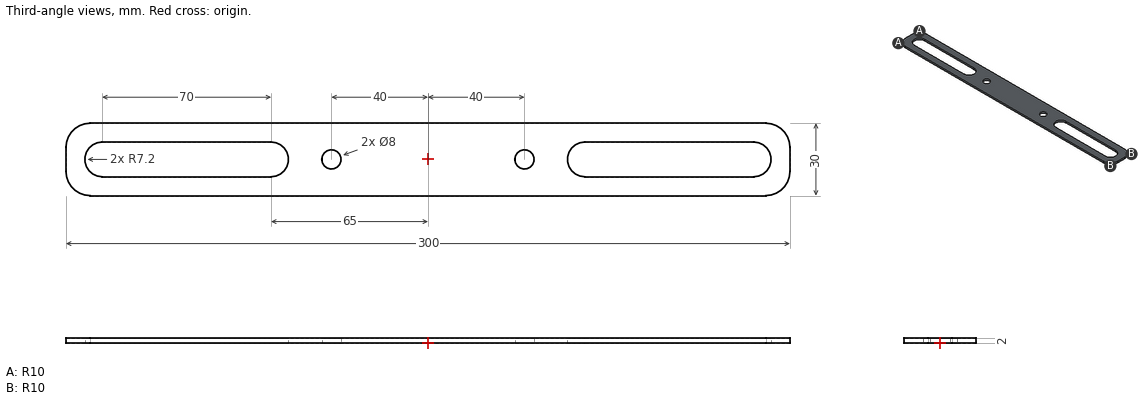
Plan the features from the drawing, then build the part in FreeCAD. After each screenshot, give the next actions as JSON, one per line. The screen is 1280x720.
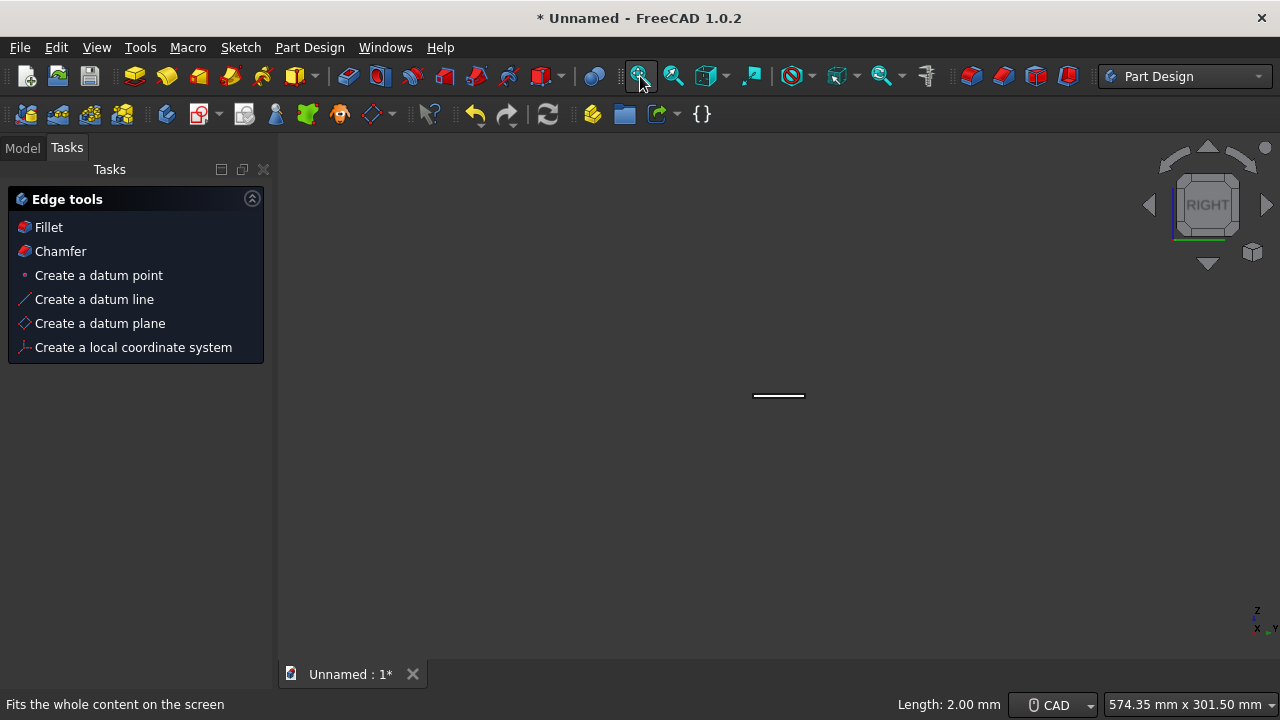
{"action": "scroll", "coordinate": [805, 395], "scroll_direction": "up", "scroll_amount": 13}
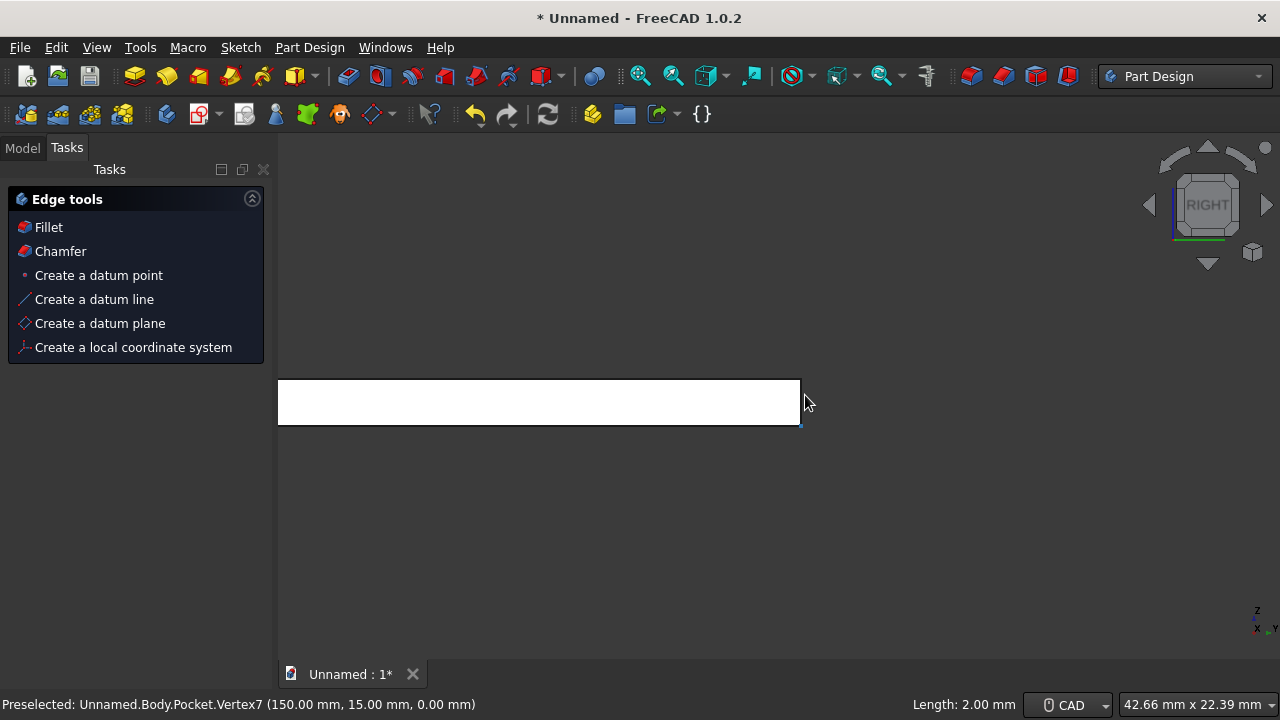
{"action": "key", "text": "v f"}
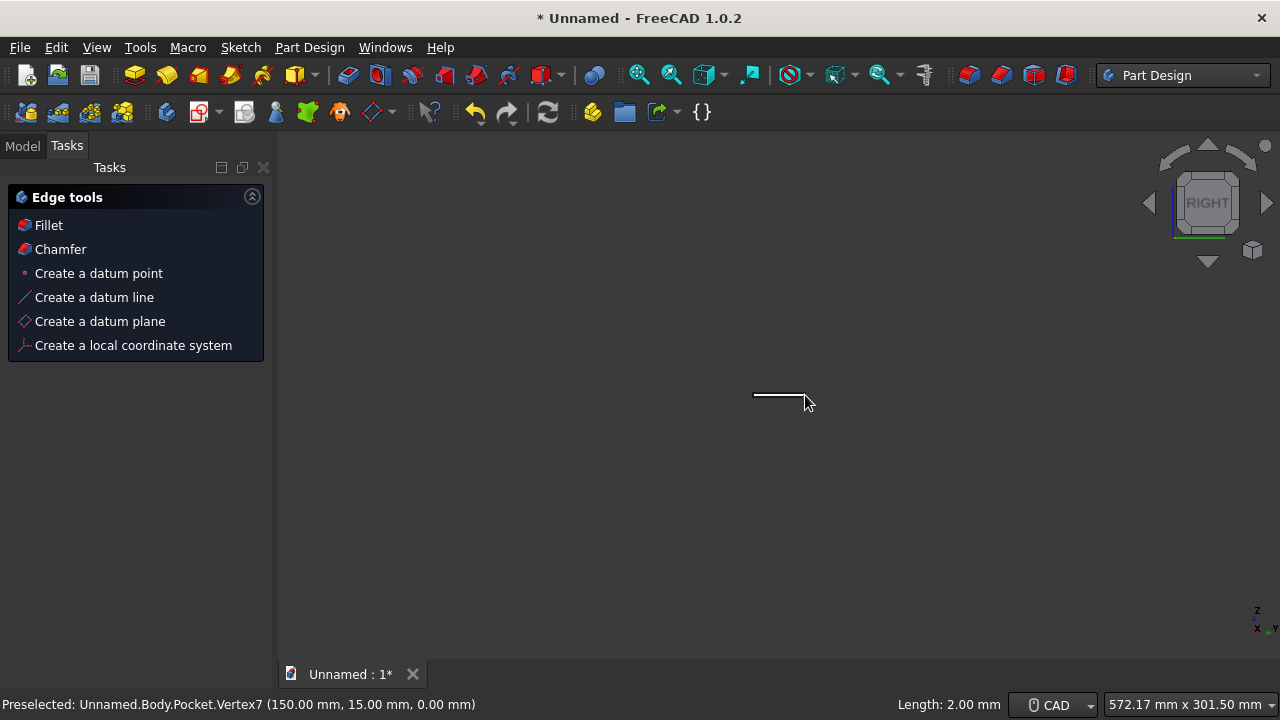
{"action": "key", "text": "5"}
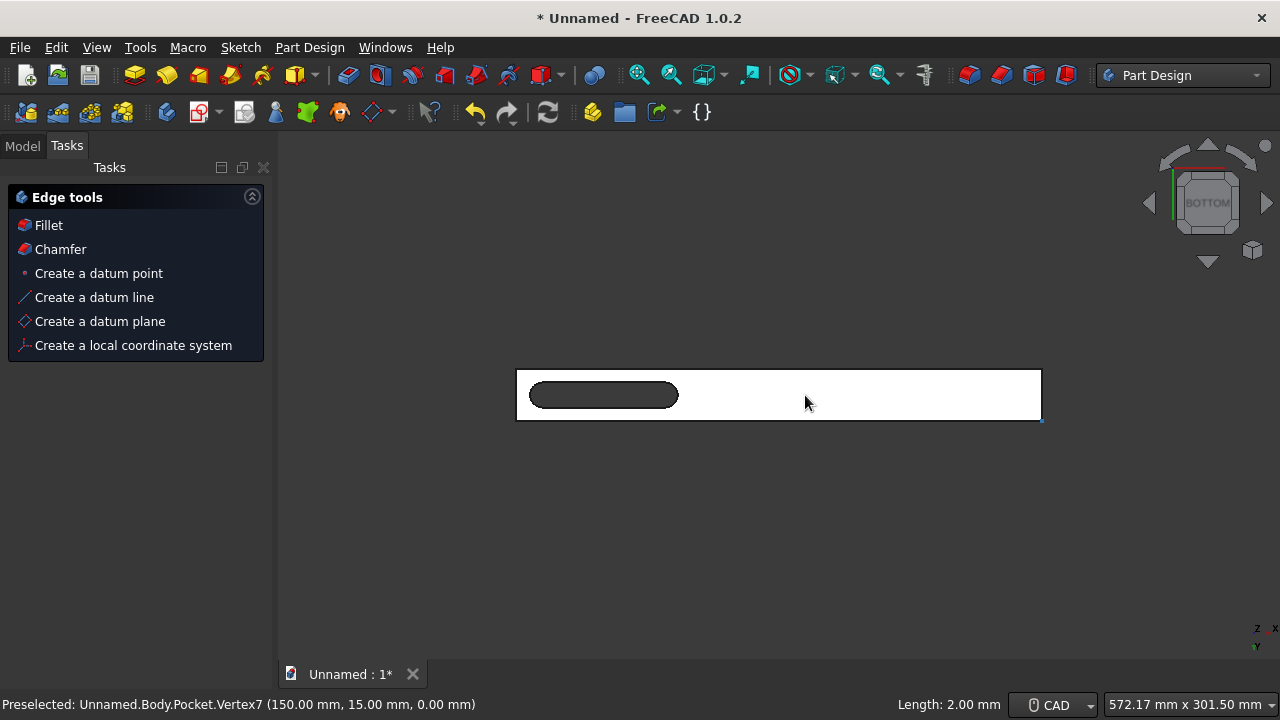
{"action": "scroll", "coordinate": [516, 420], "scroll_direction": "up", "scroll_amount": 13}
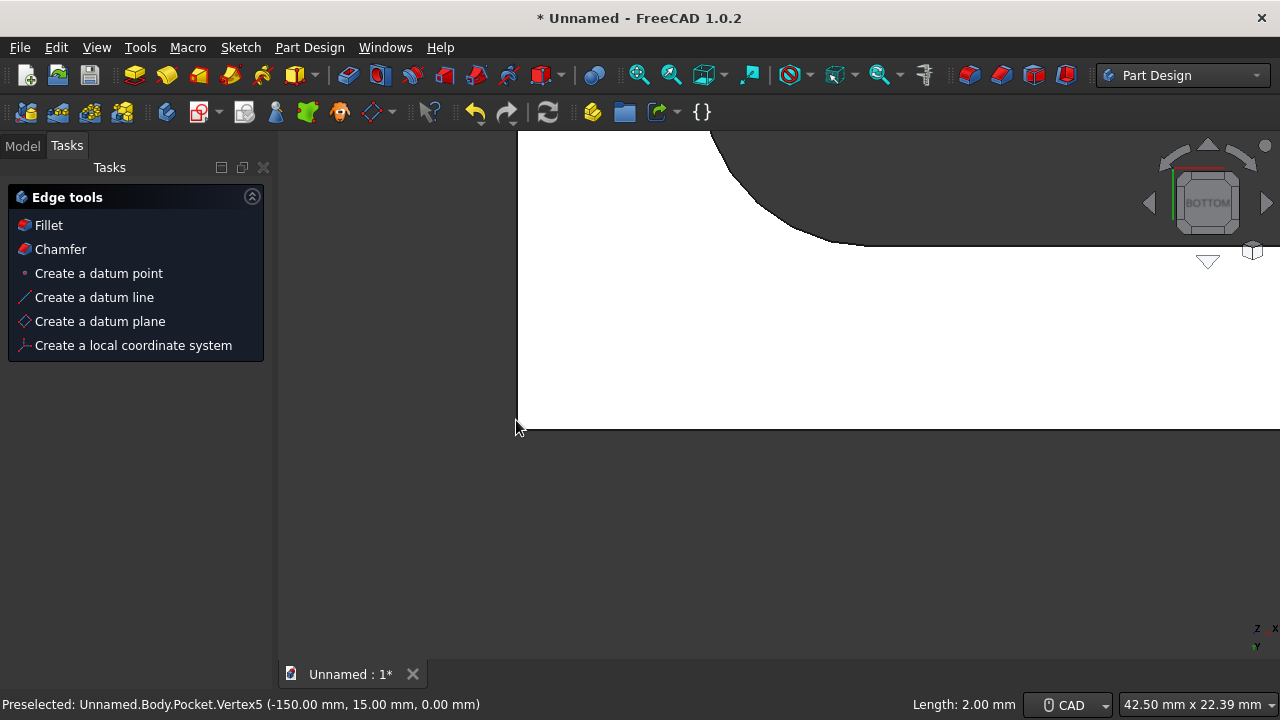
{"action": "key", "text": "v f"}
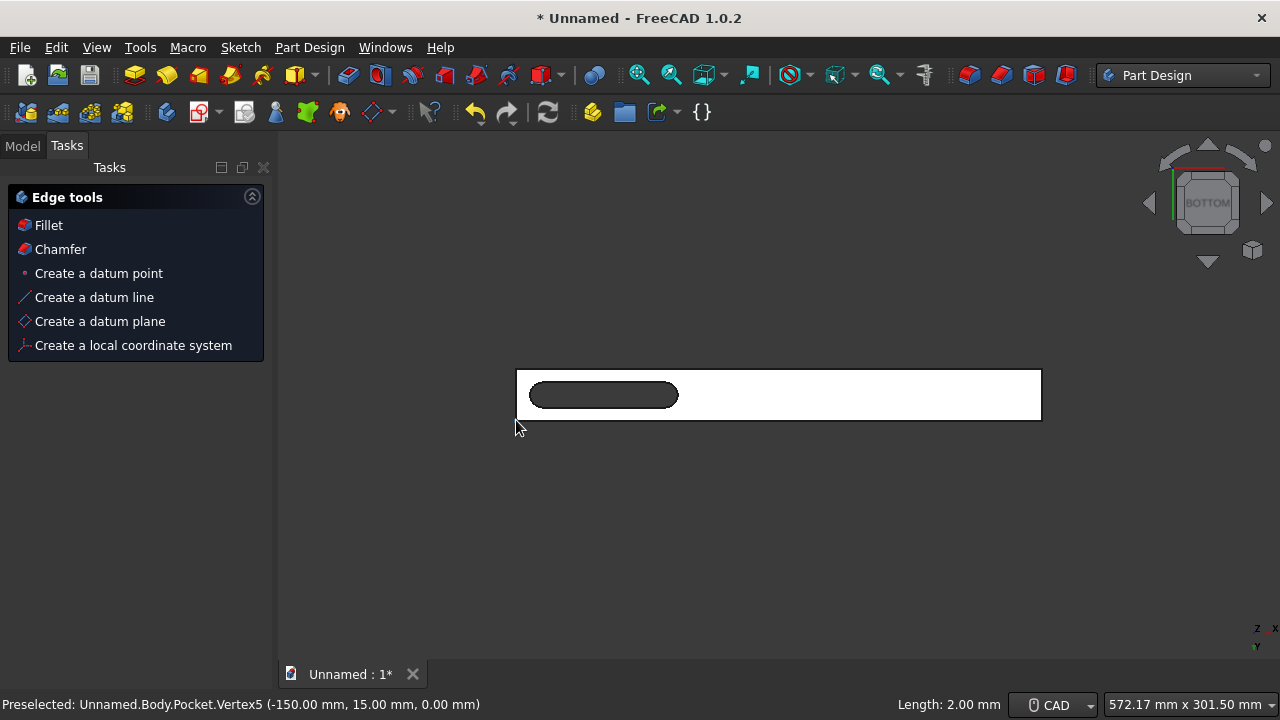
{"action": "key", "text": "4"}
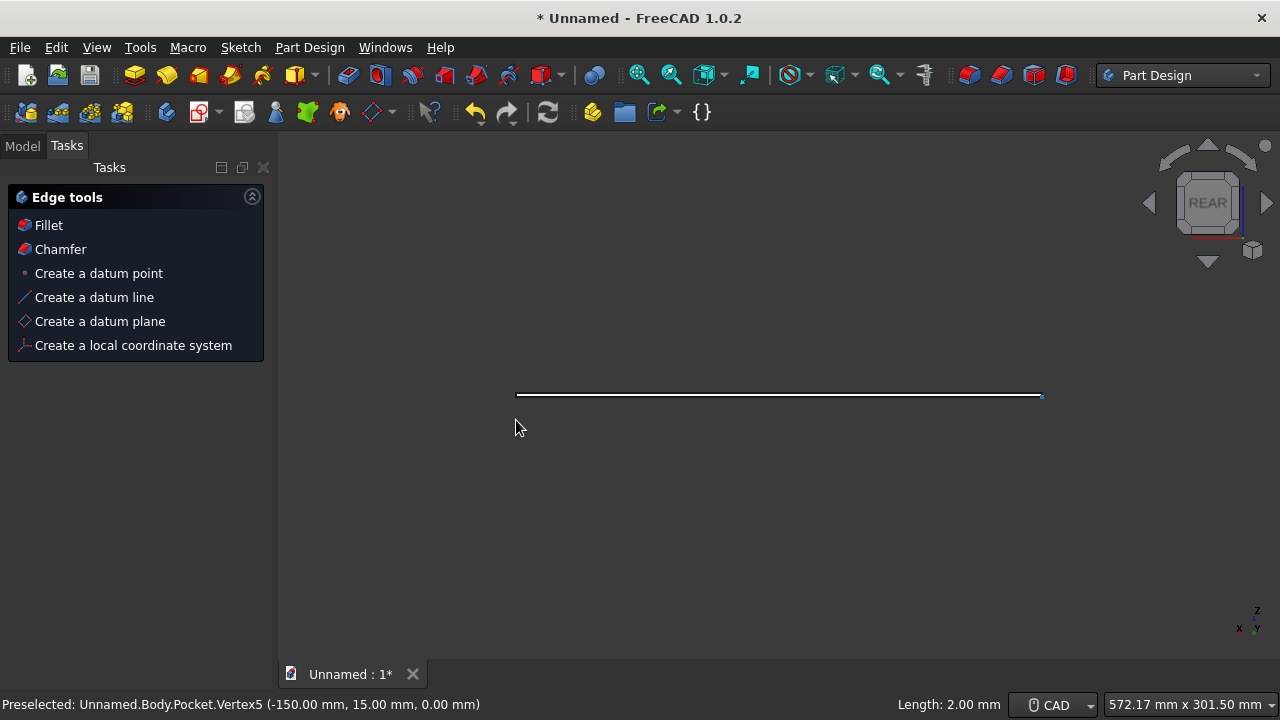
{"action": "scroll", "coordinate": [1042, 394], "scroll_direction": "up", "scroll_amount": 13}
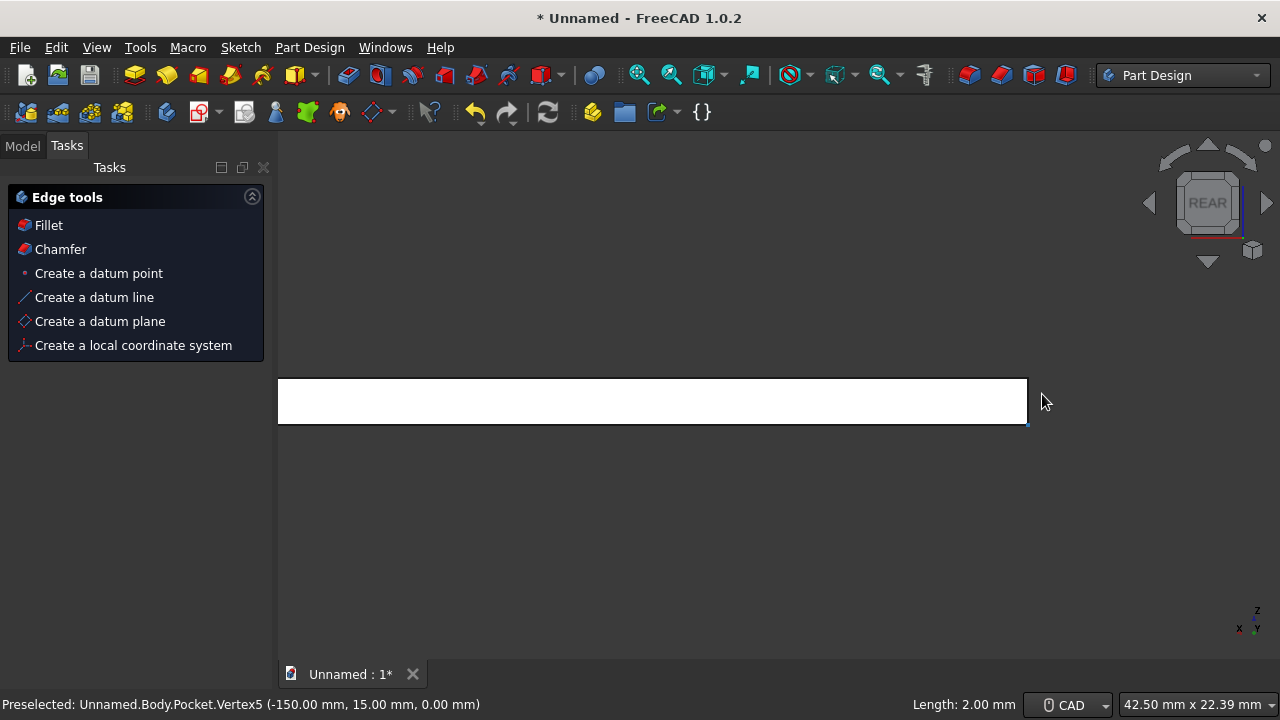
{"action": "left_click", "coordinate": [1028, 400], "text": "ctrl"}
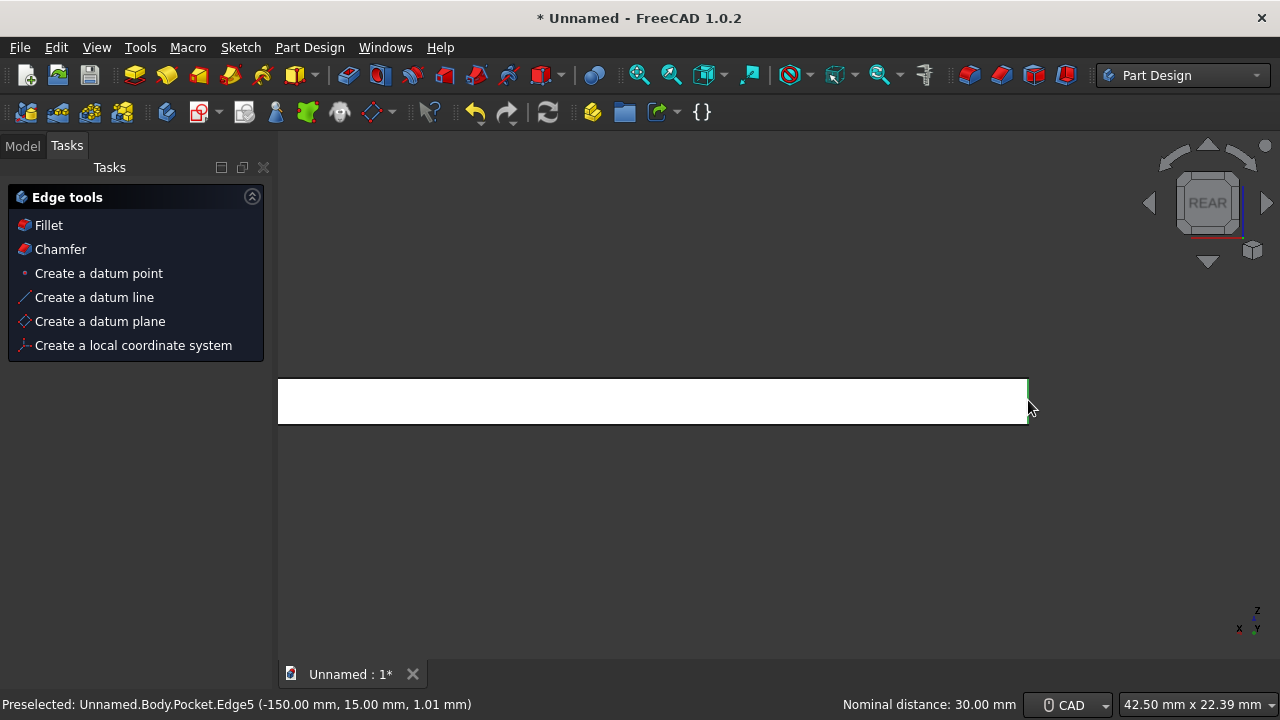
{"action": "left_click", "coordinate": [970, 76]}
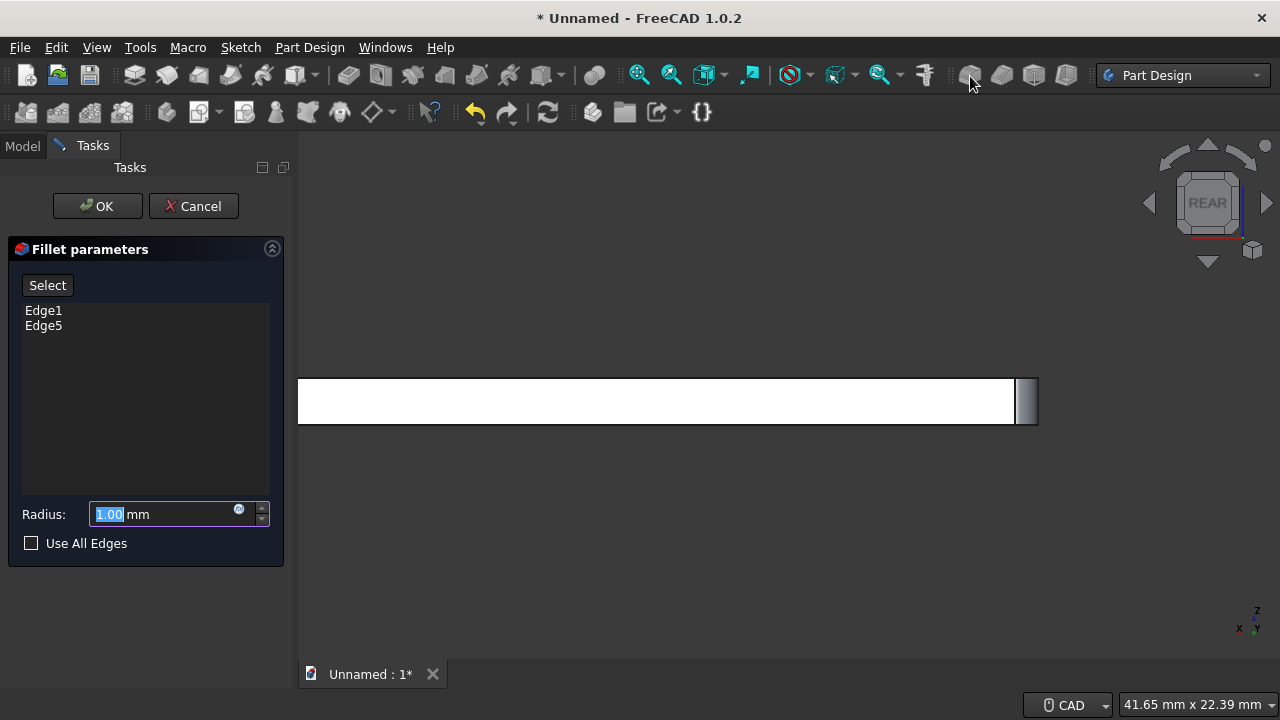
{"action": "type", "text": "10"}
{"action": "key", "text": "Tab"}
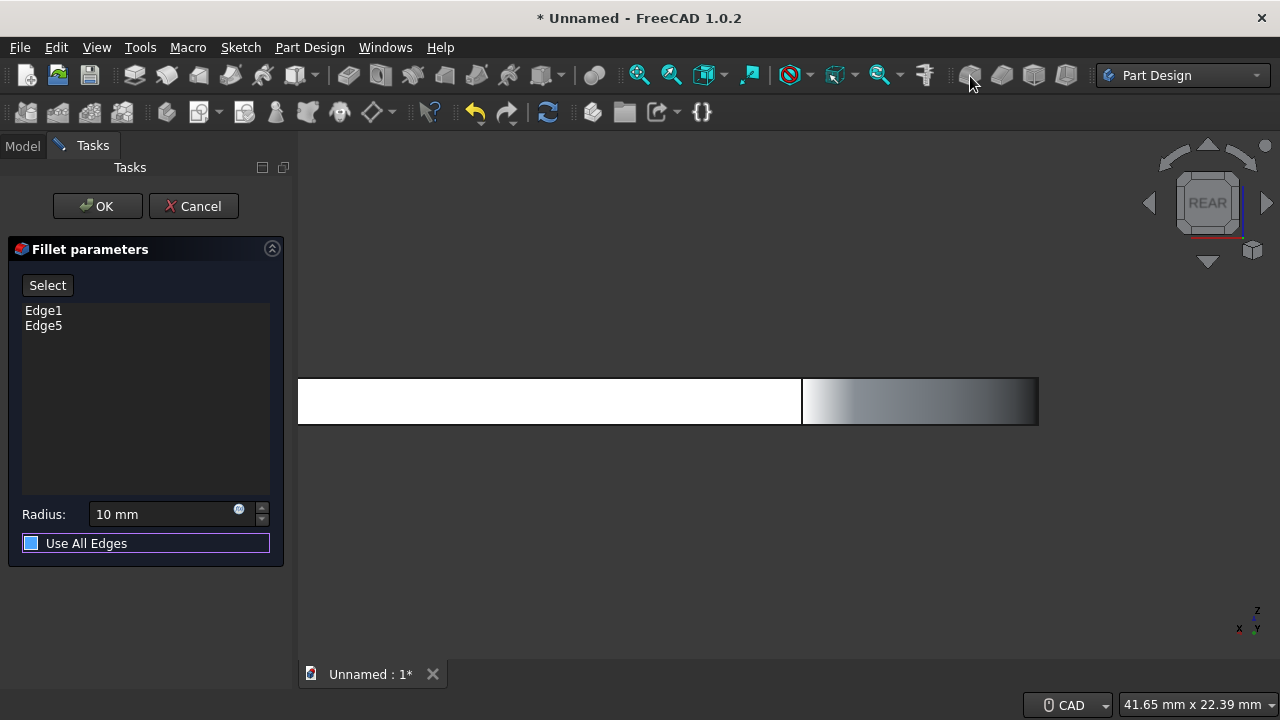
{"action": "left_click", "coordinate": [98, 206]}